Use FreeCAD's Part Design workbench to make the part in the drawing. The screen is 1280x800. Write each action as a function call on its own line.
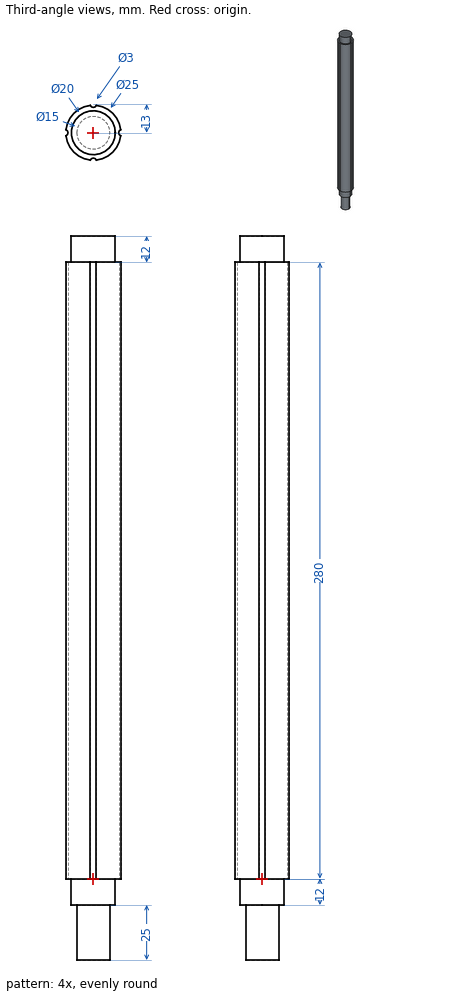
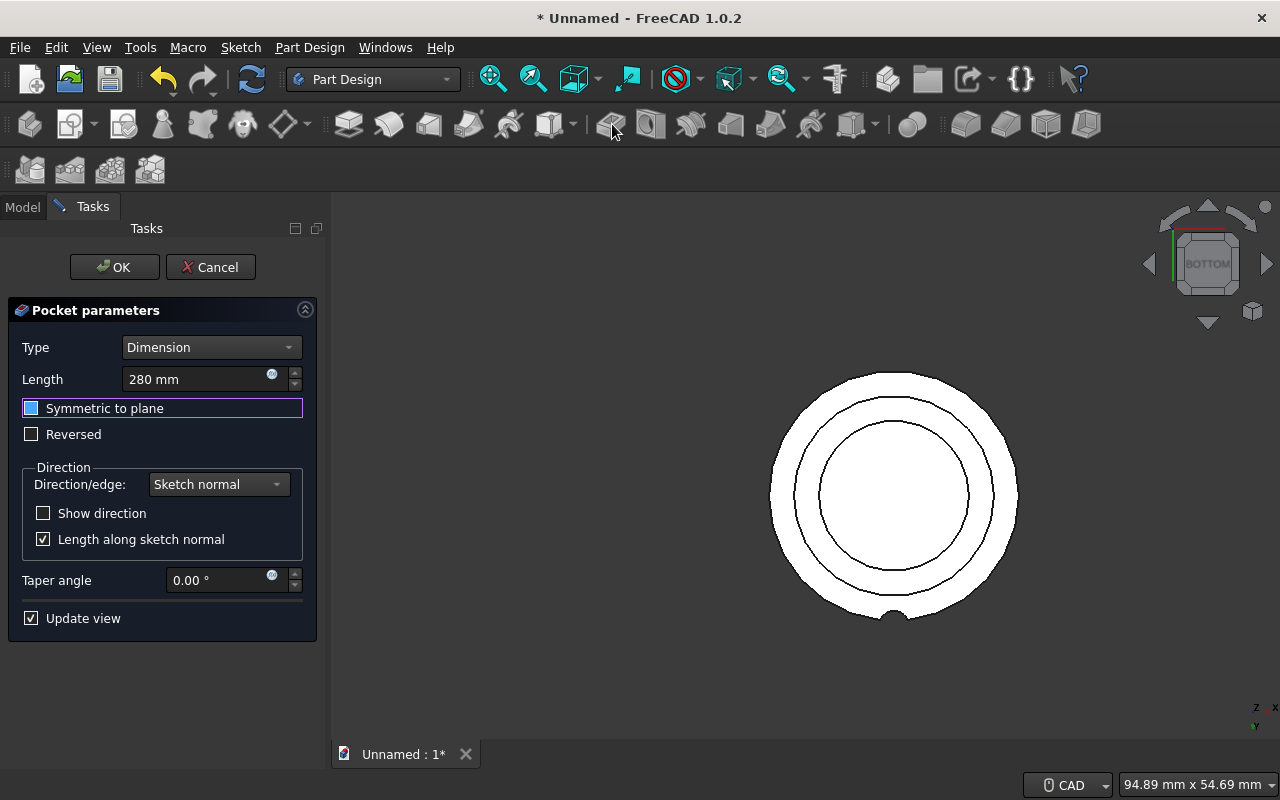
click(115, 267)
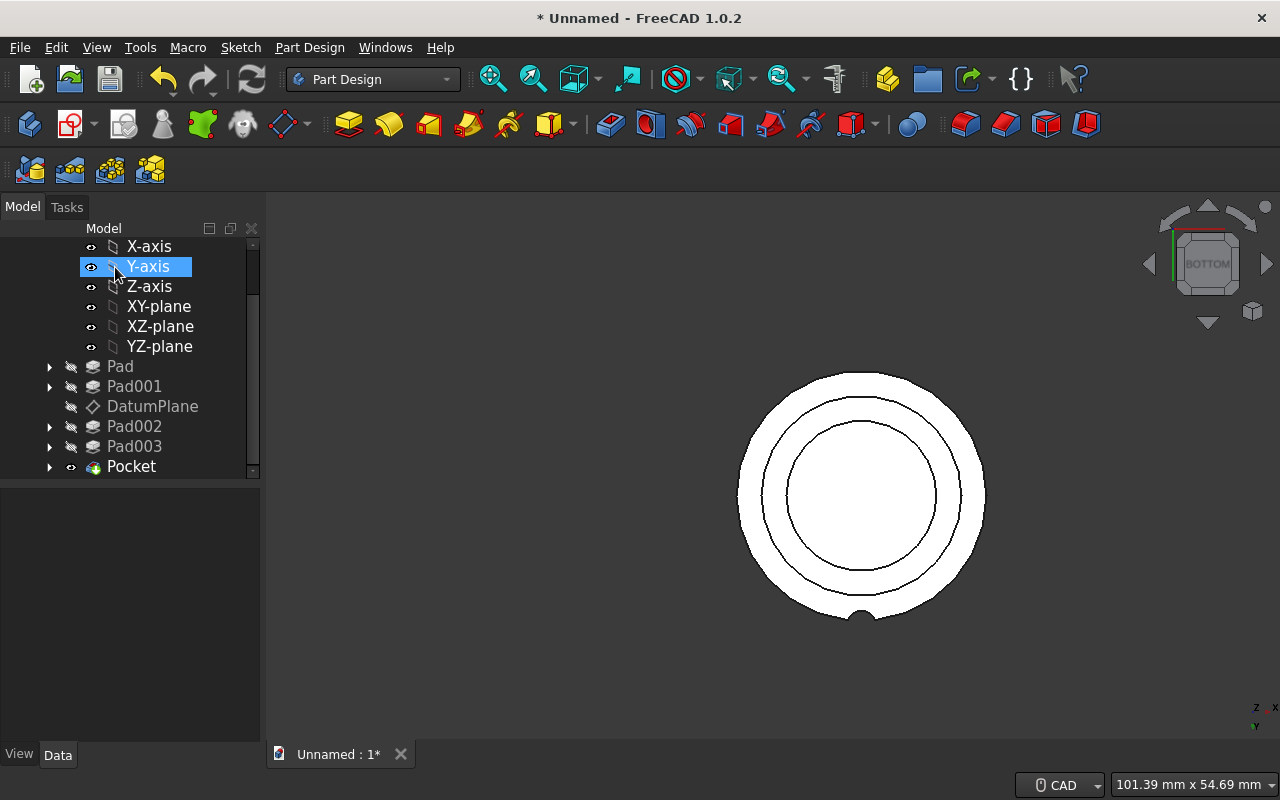
click(116, 467)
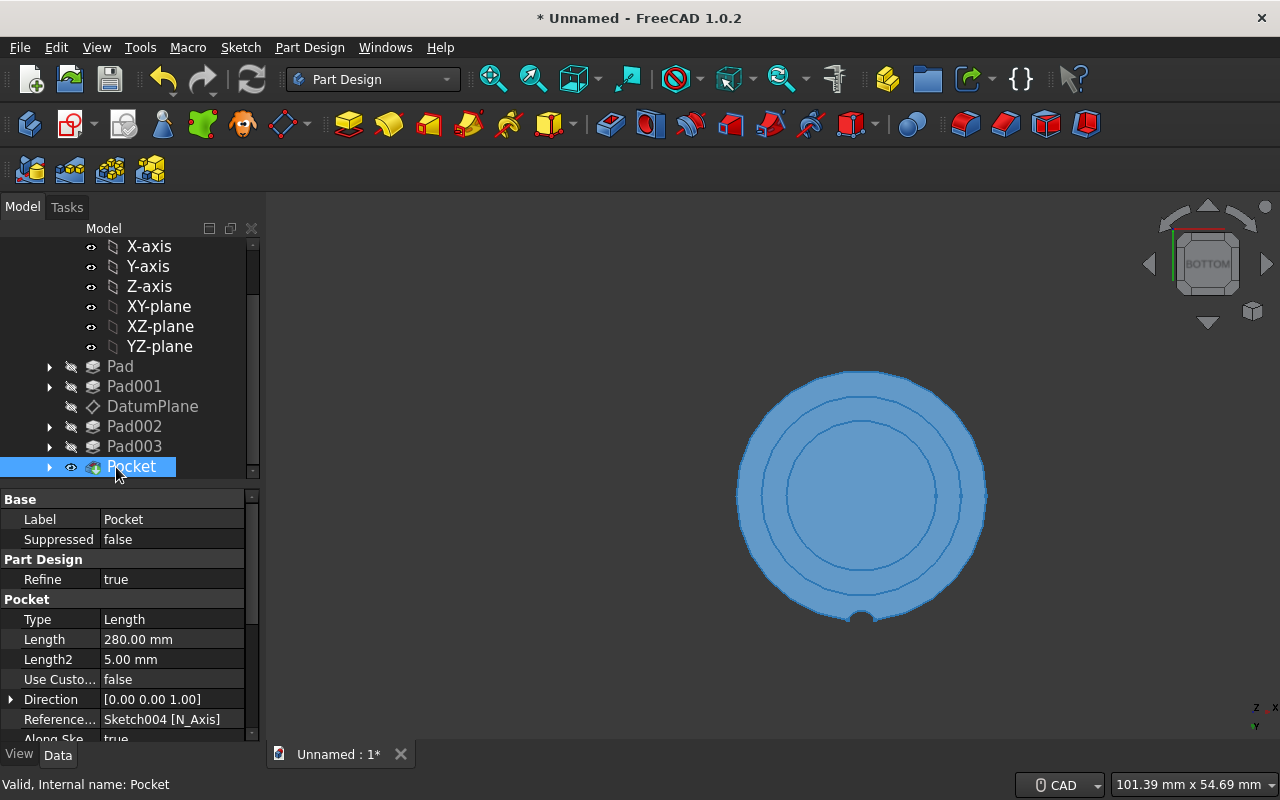
click(110, 170)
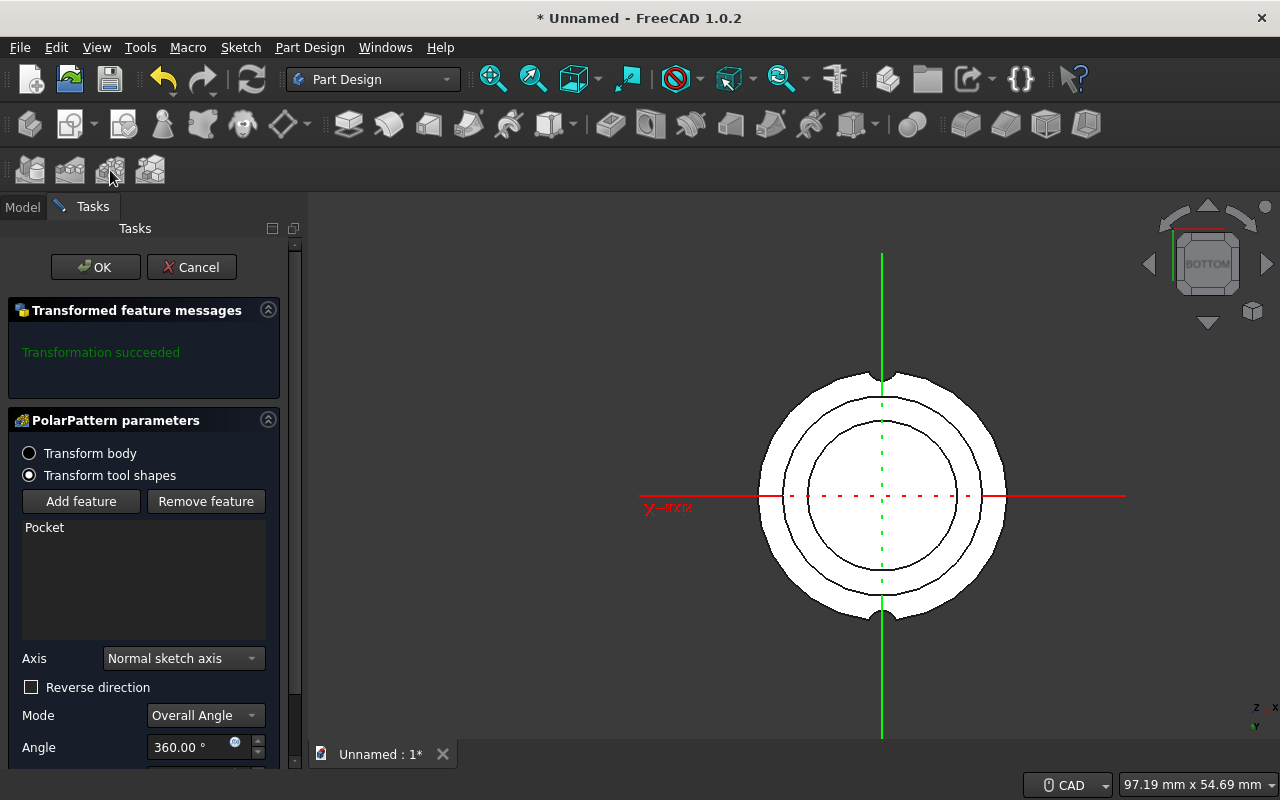
click(184, 658)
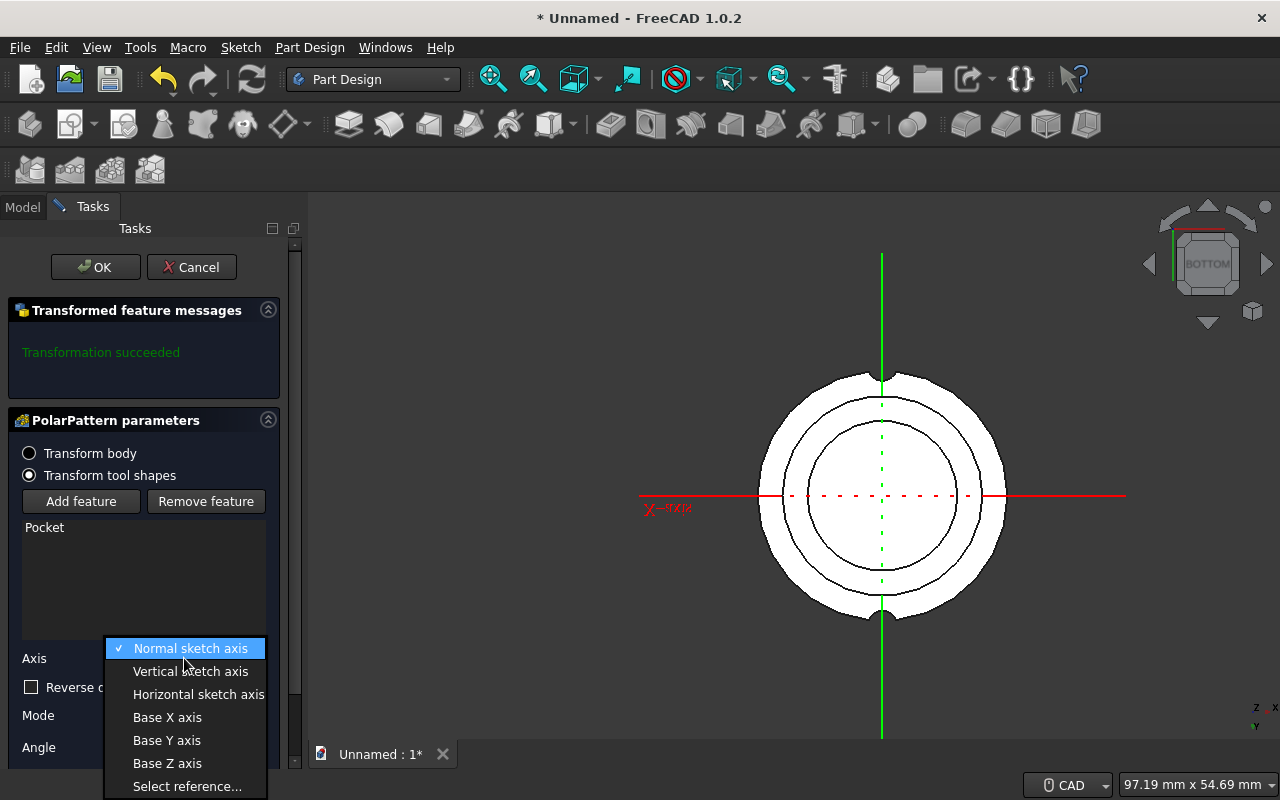
click(184, 764)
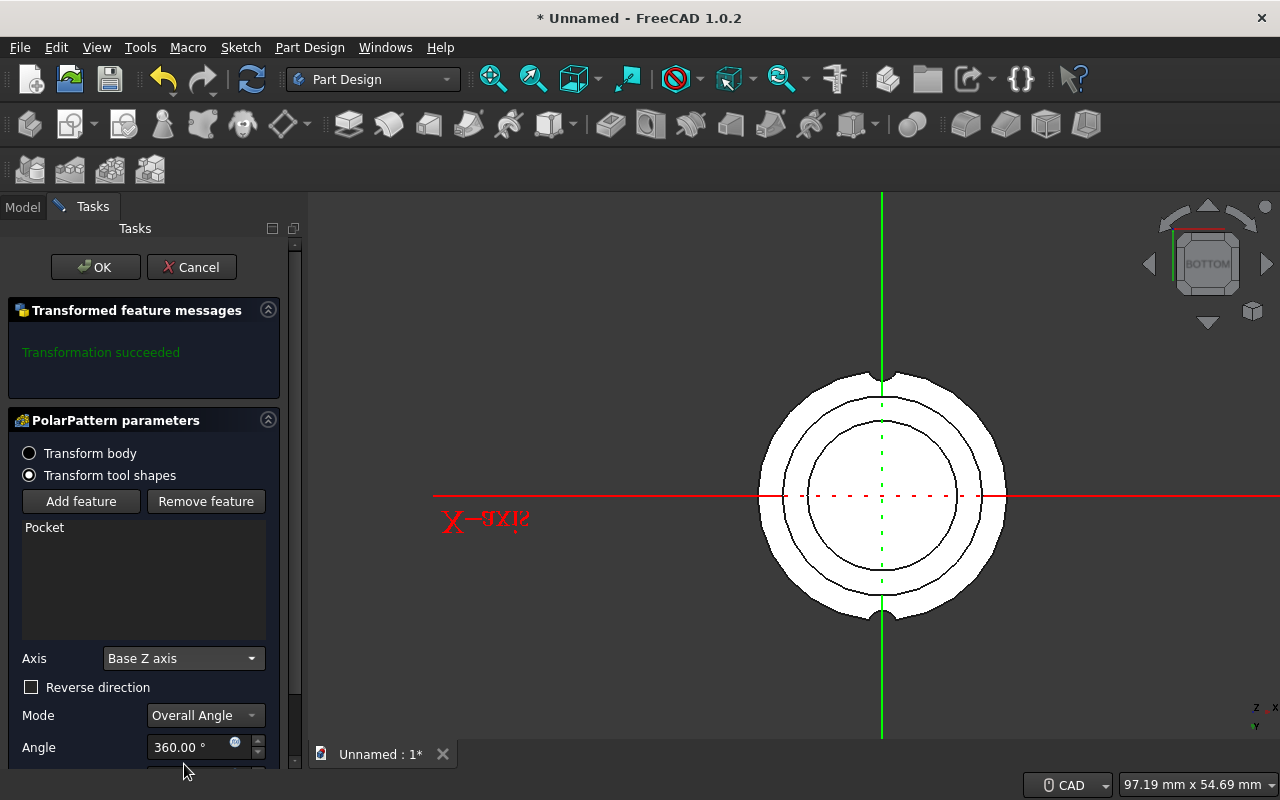
scroll(295, 503, down, 2)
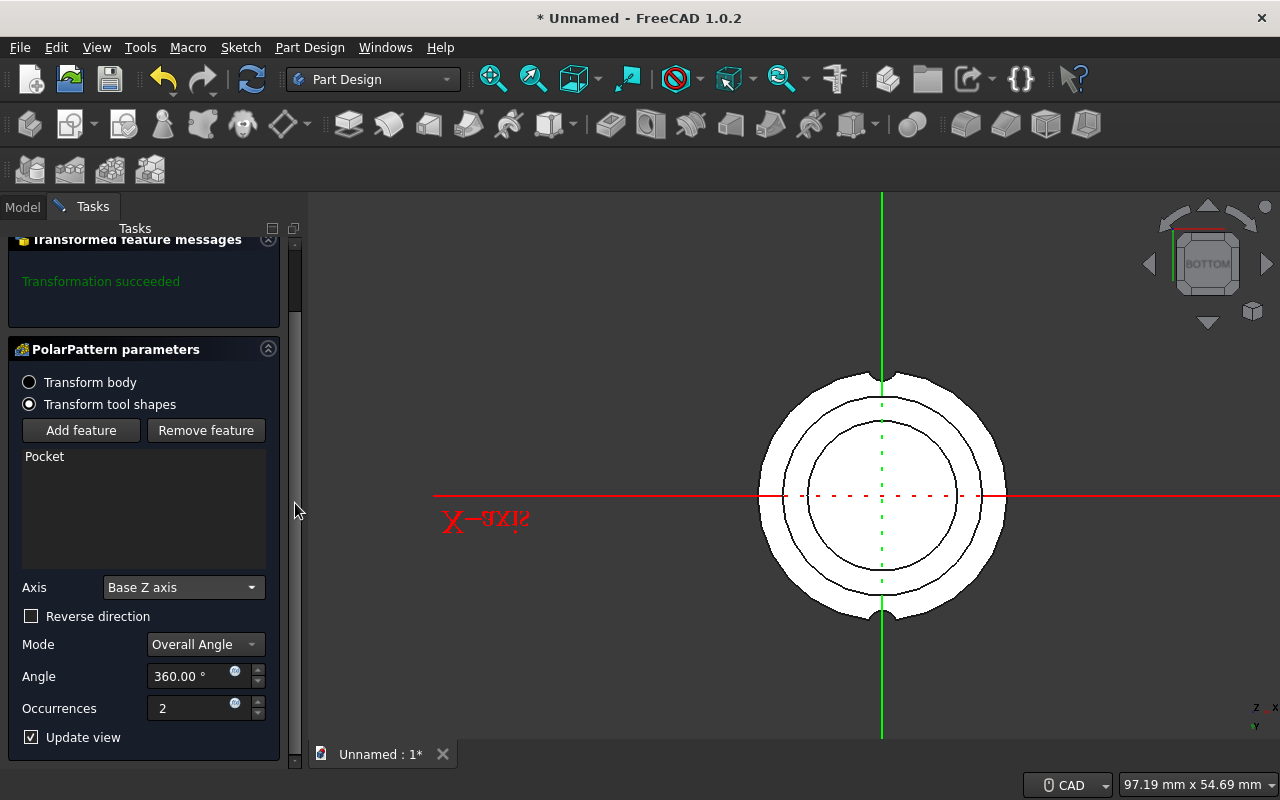
triple_click(198, 708)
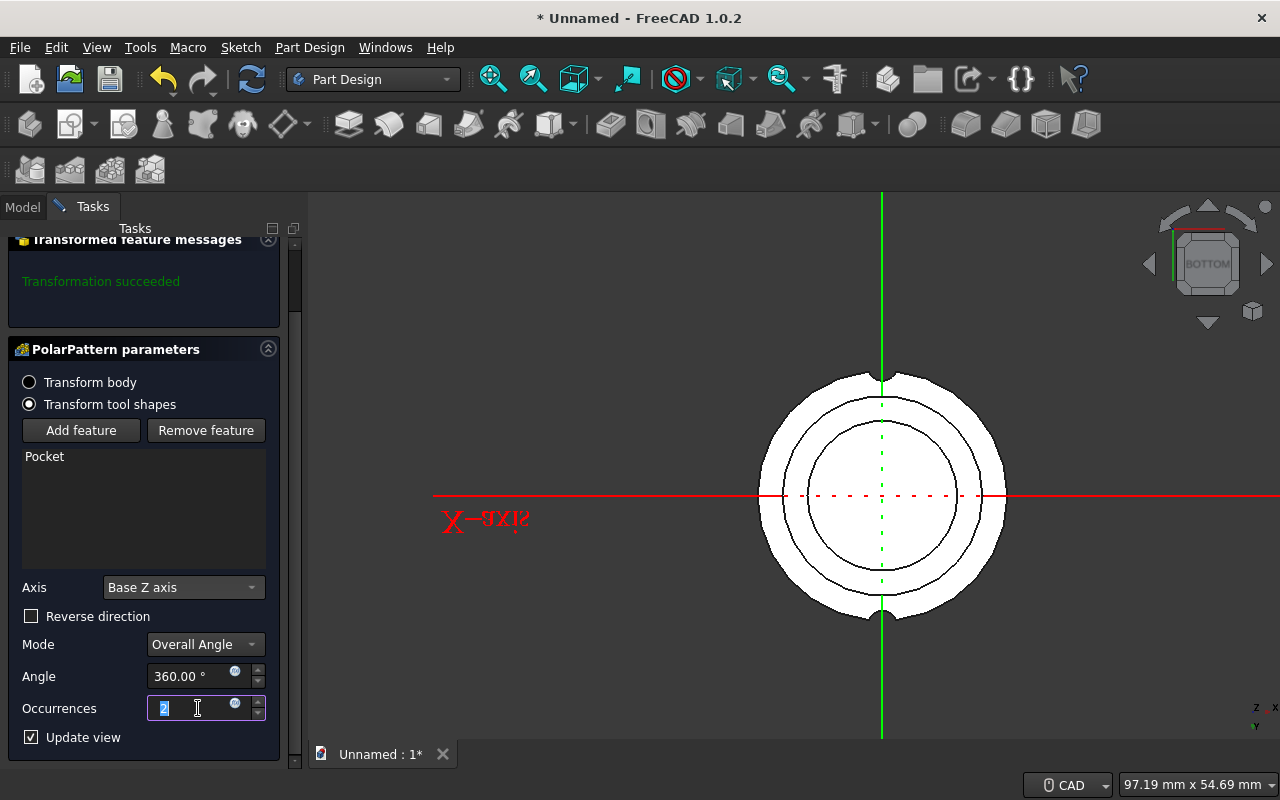
text(4)
key(Tab)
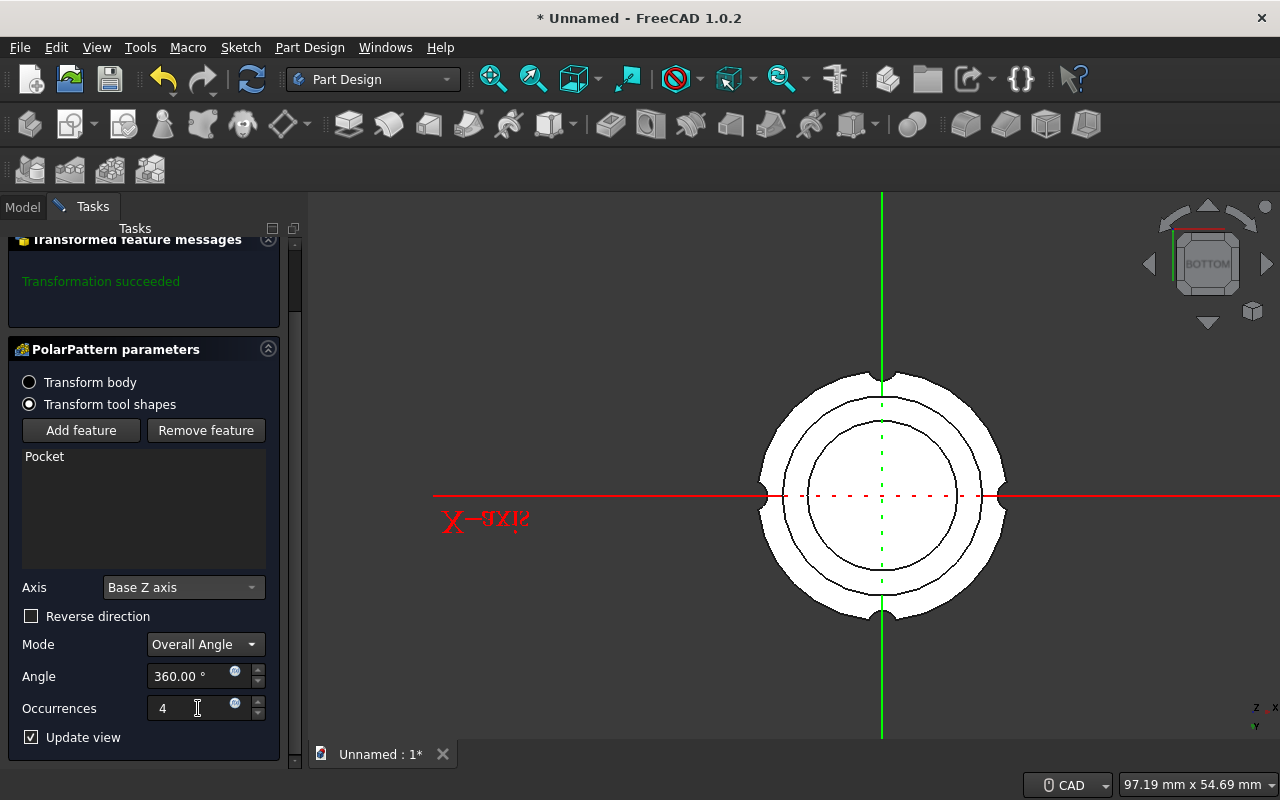
scroll(295, 503, up, 2)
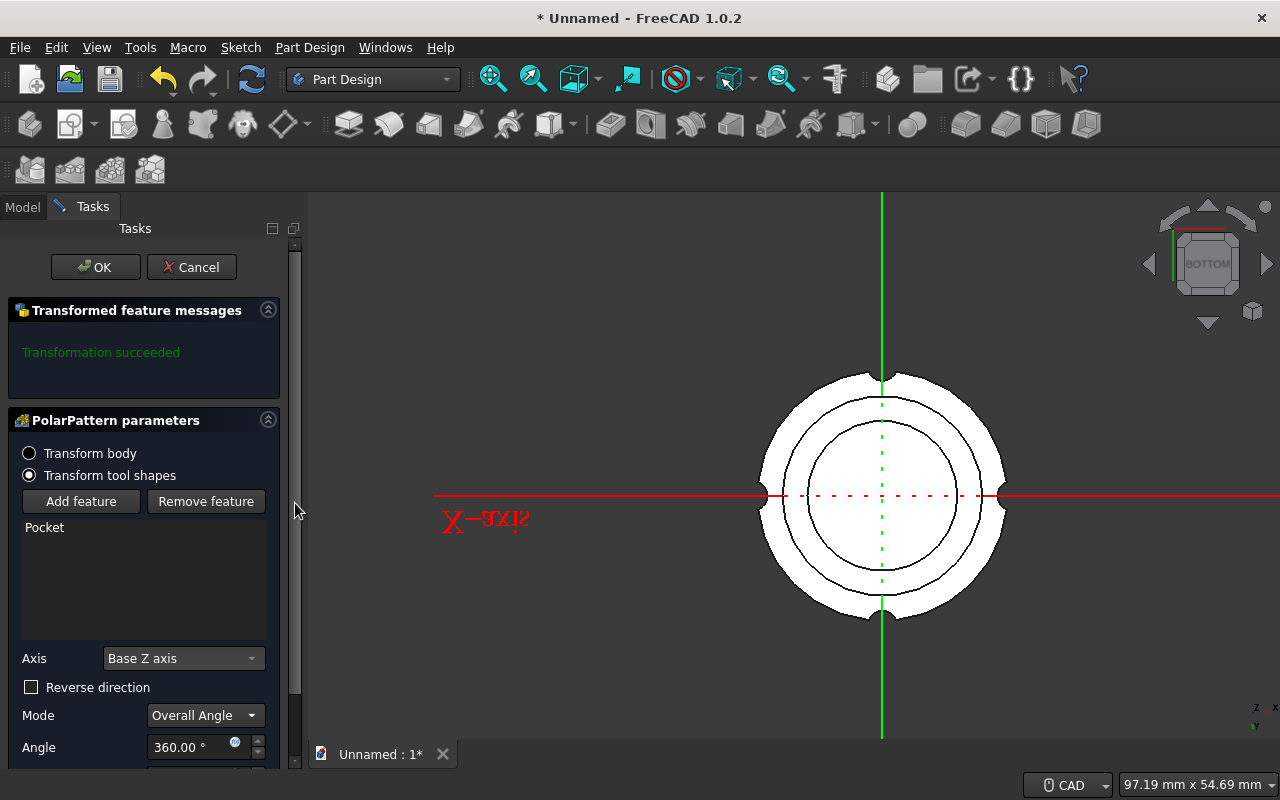
click(96, 267)